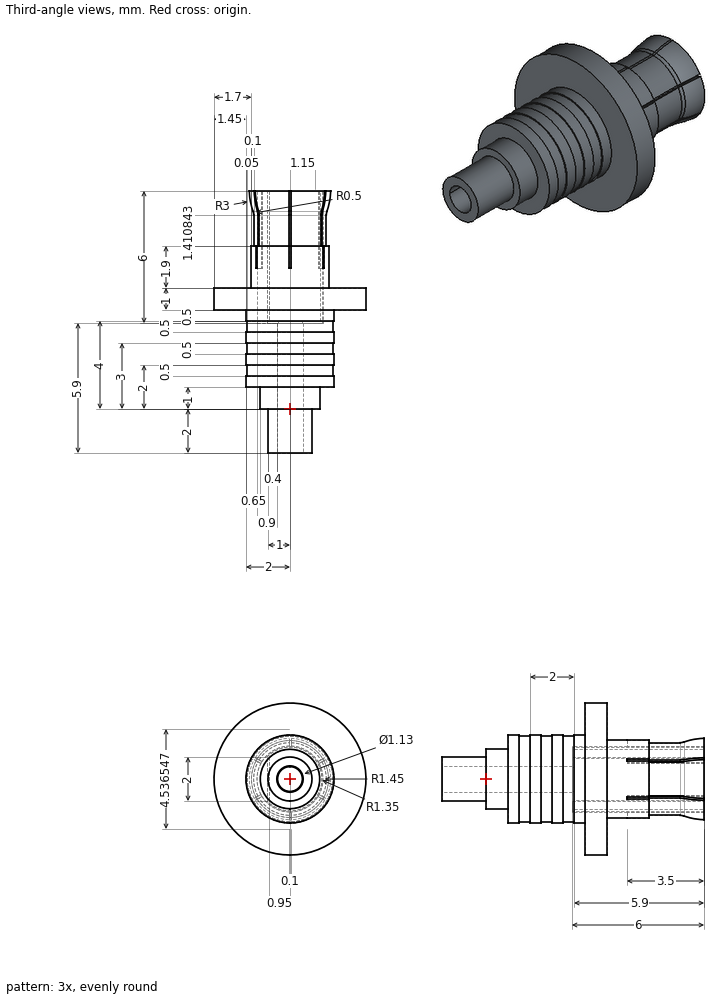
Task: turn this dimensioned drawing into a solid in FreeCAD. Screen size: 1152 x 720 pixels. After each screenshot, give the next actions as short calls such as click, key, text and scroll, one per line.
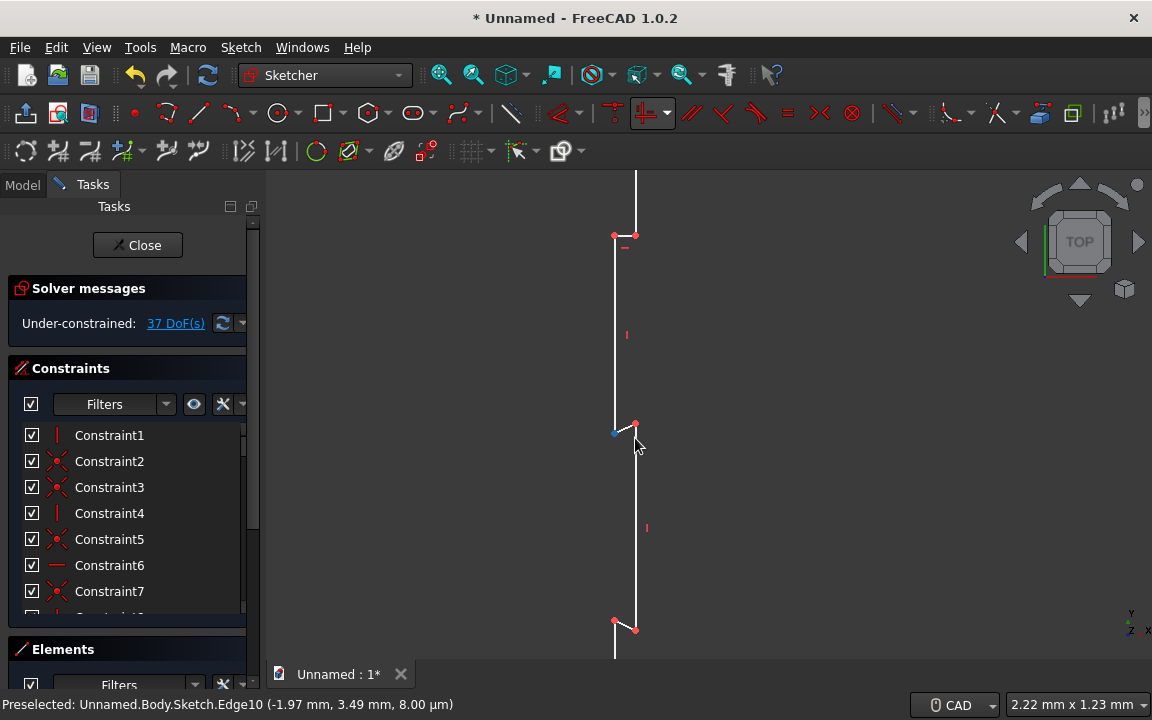
click(625, 429)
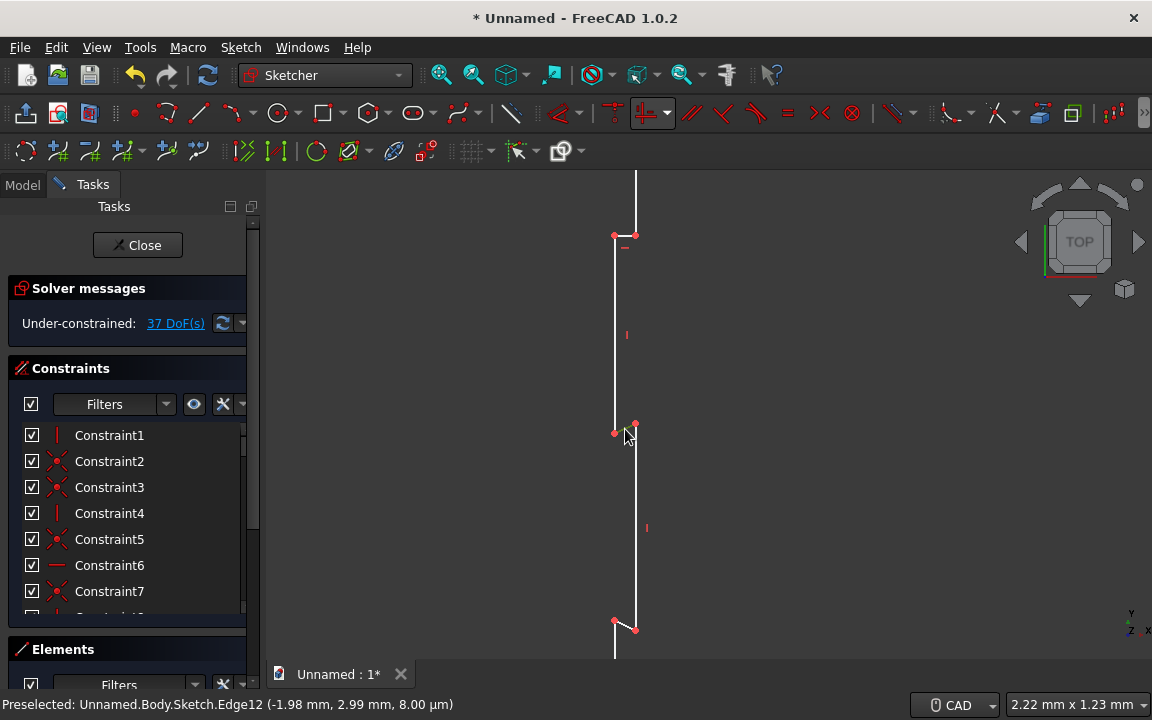
key(h)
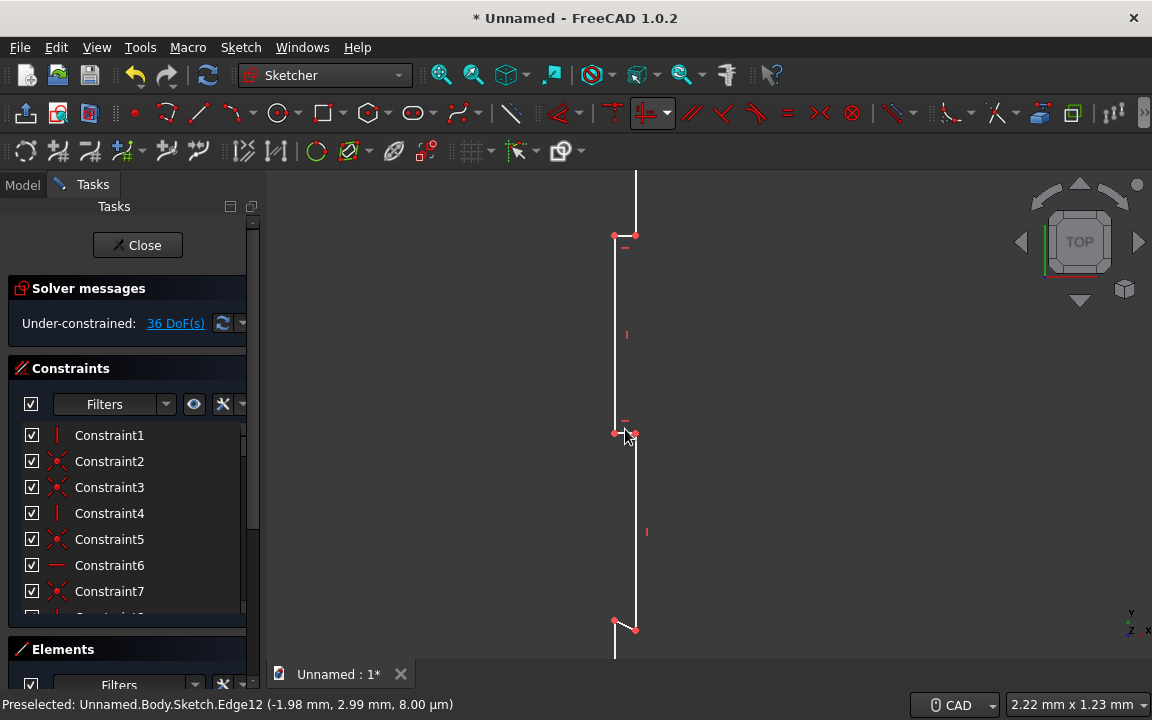
click(625, 626)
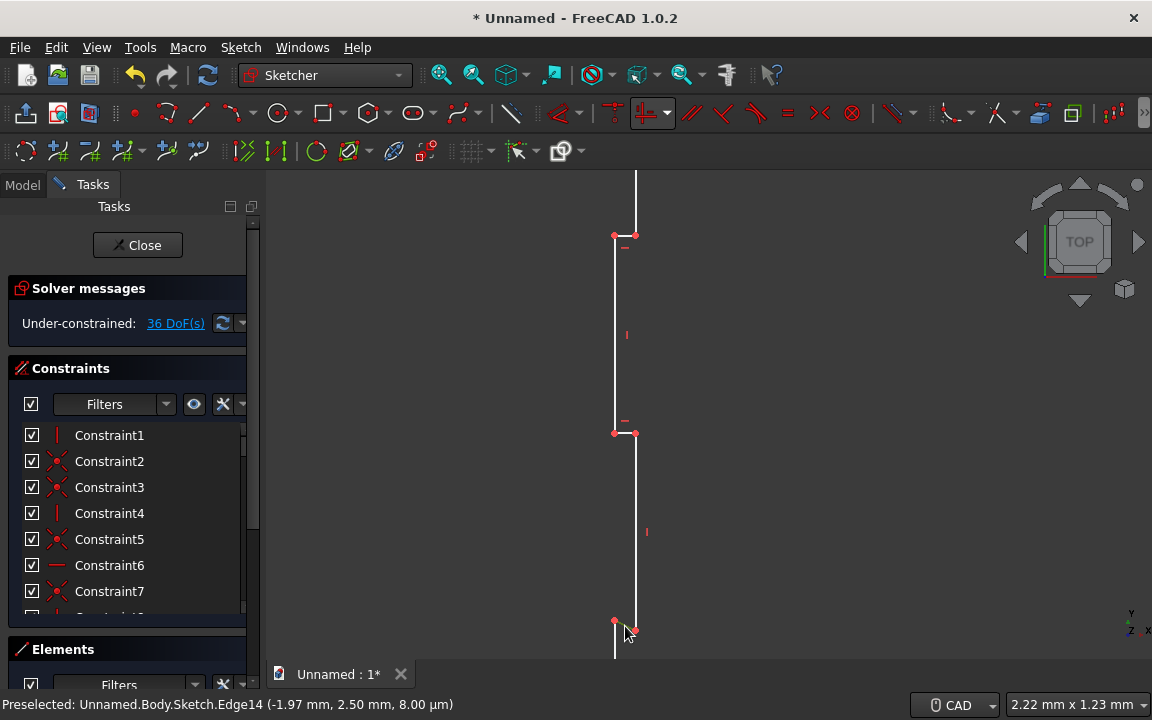
key(h)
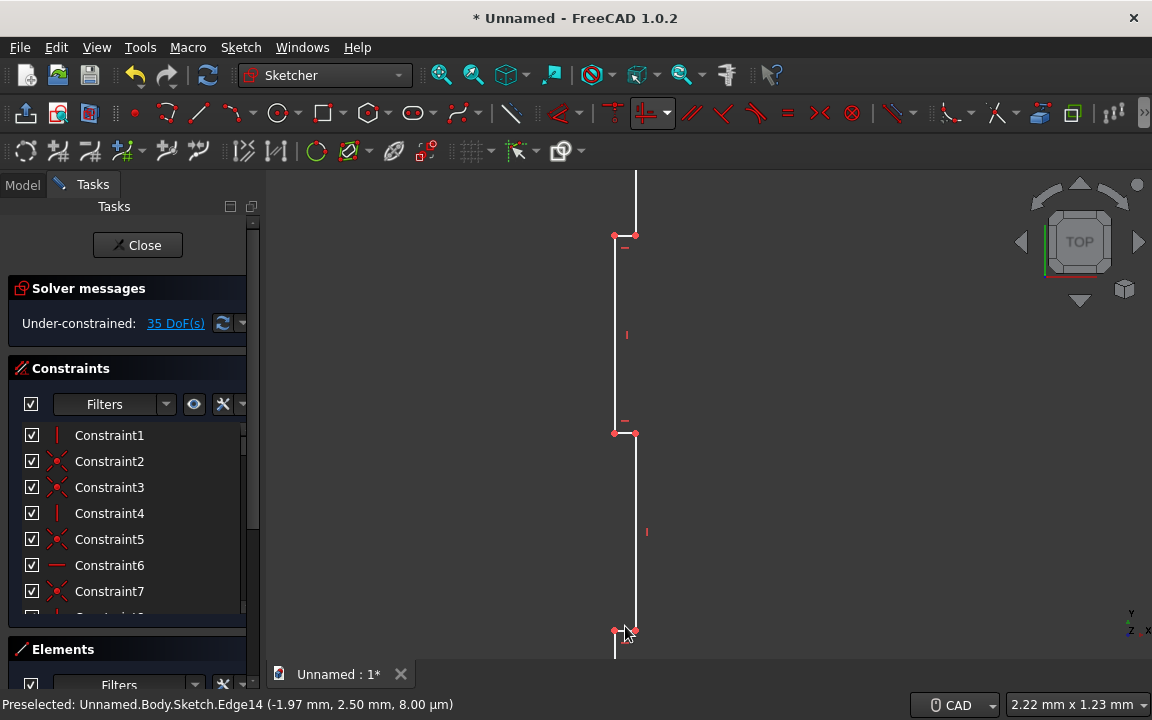
scroll(635, 438, down, 14)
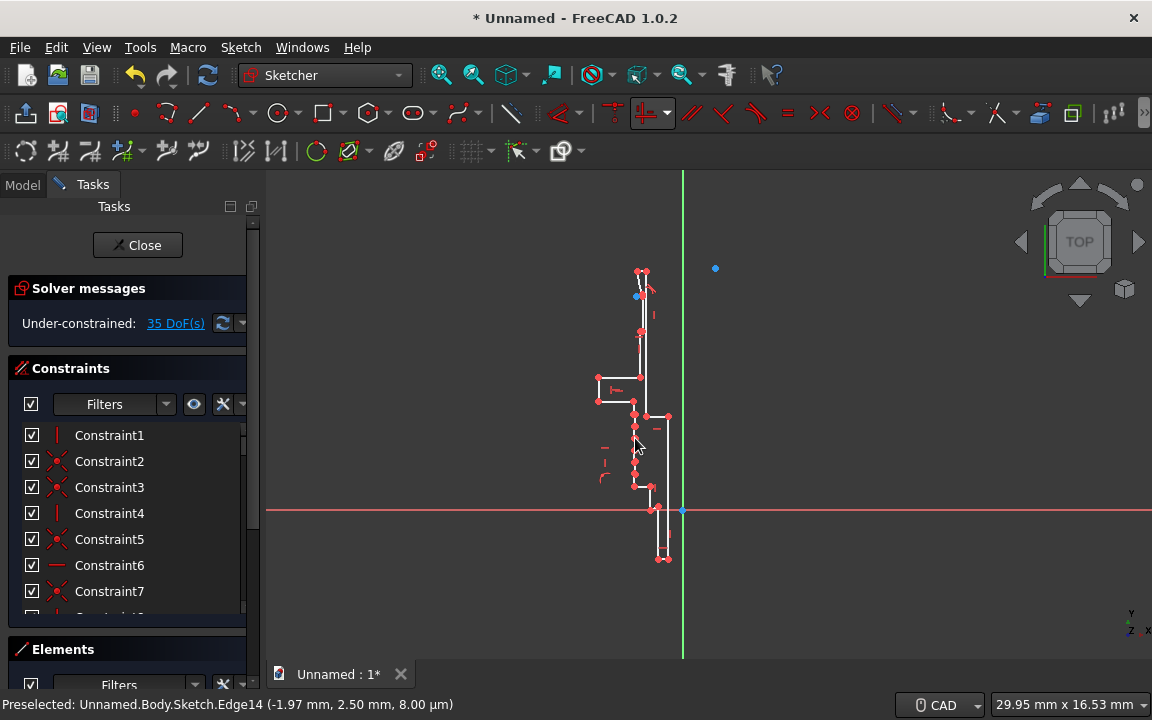
scroll(635, 462, up, 14)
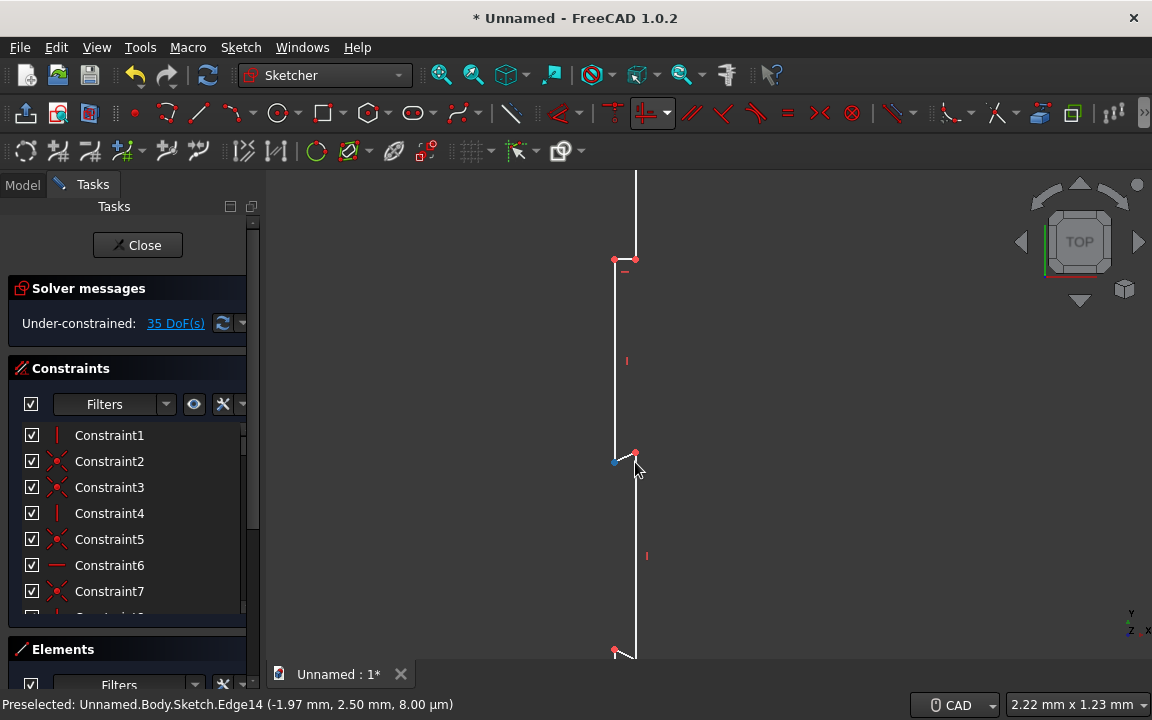
click(625, 457)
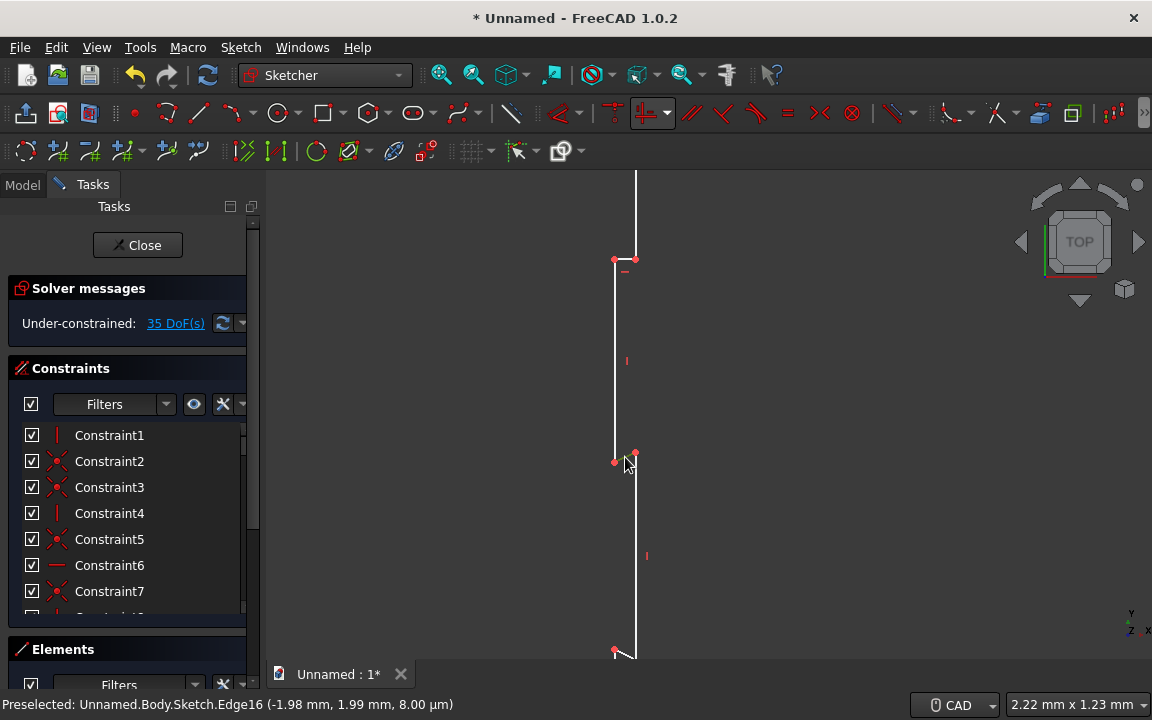
key(h)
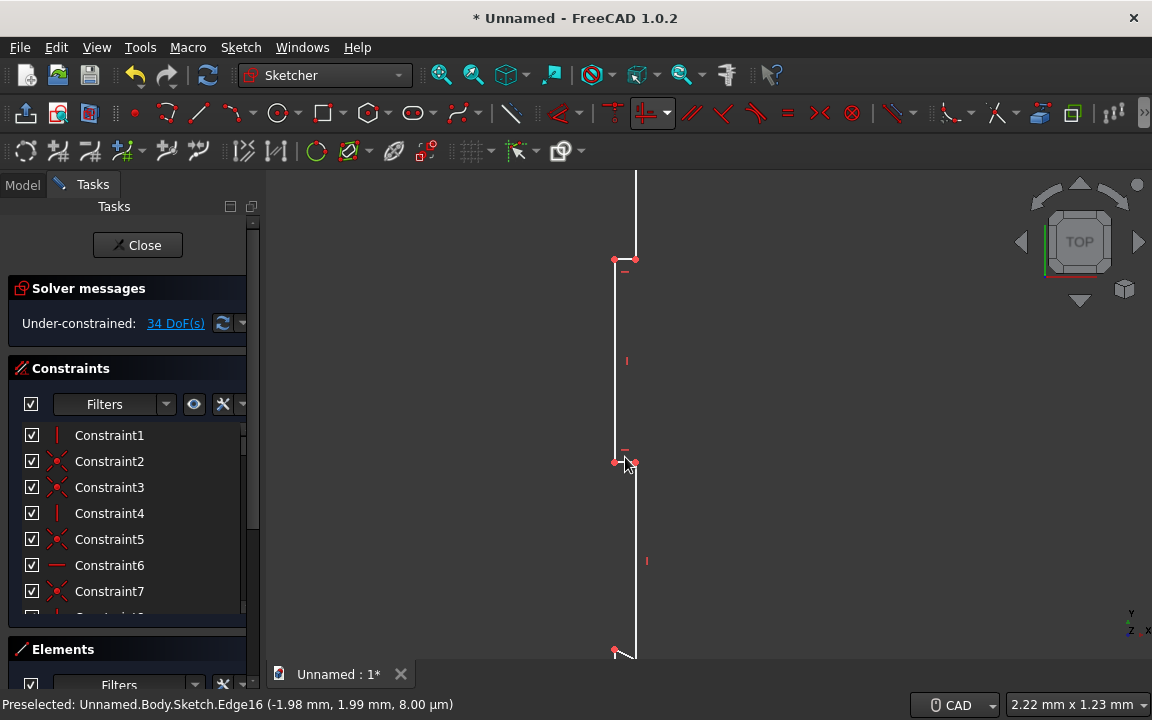
scroll(635, 462, down, 14)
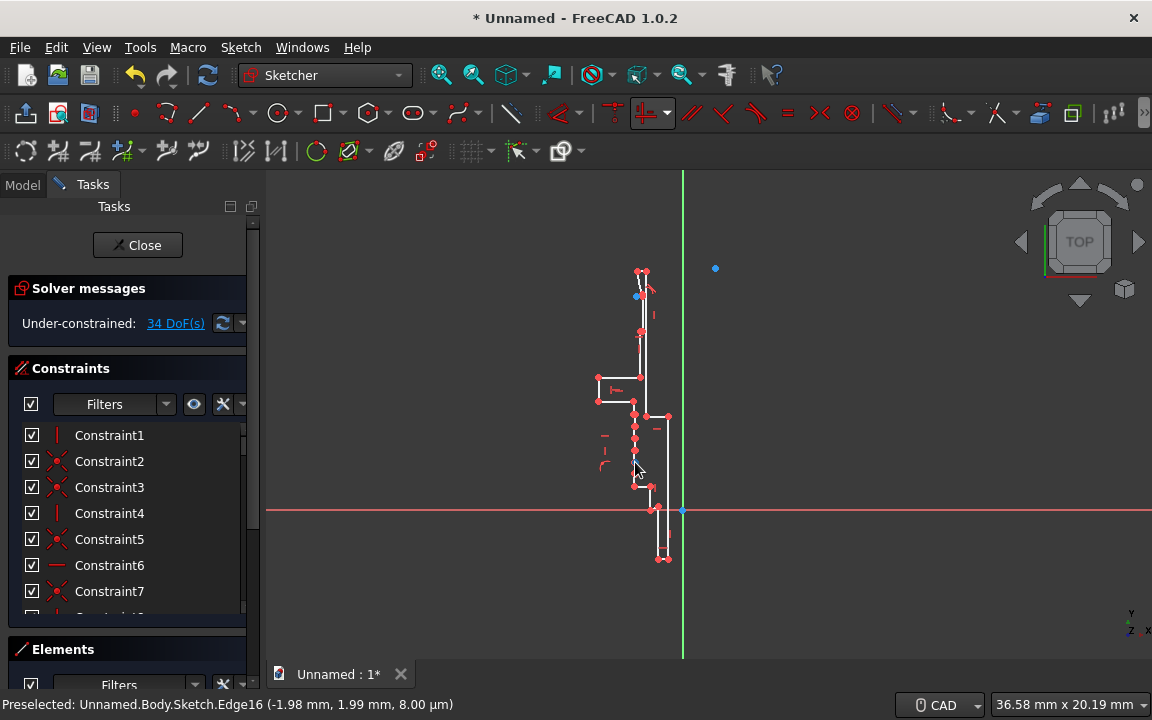
scroll(635, 474, up, 14)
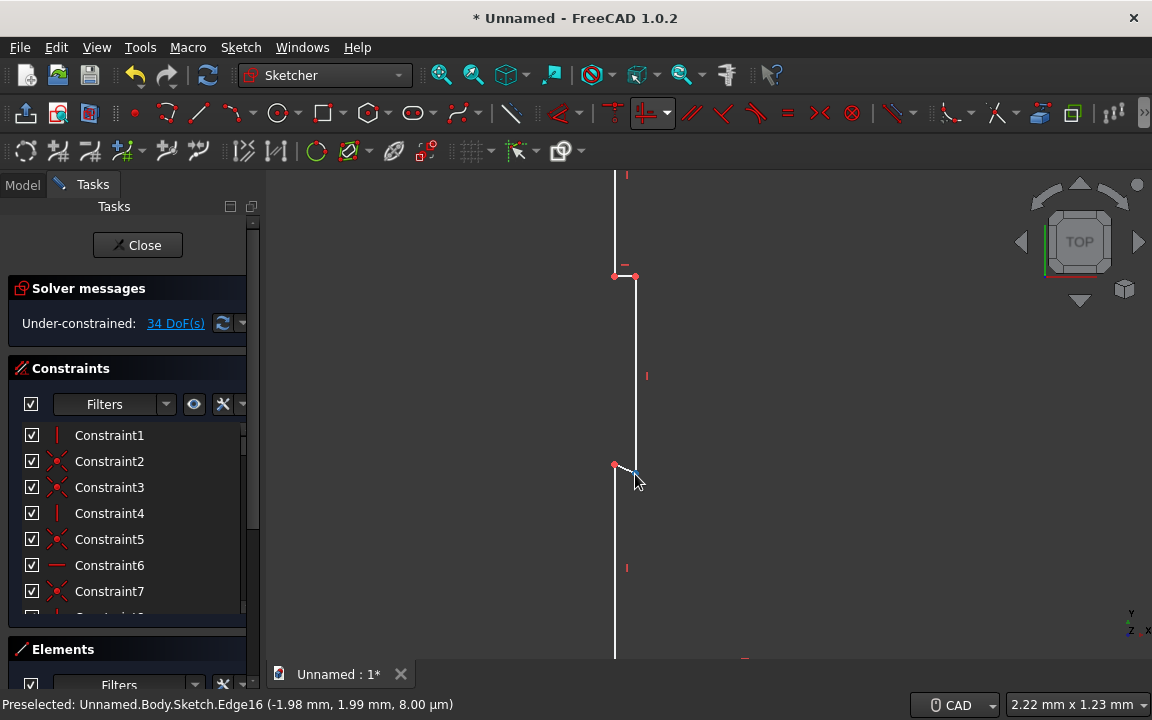
click(625, 469)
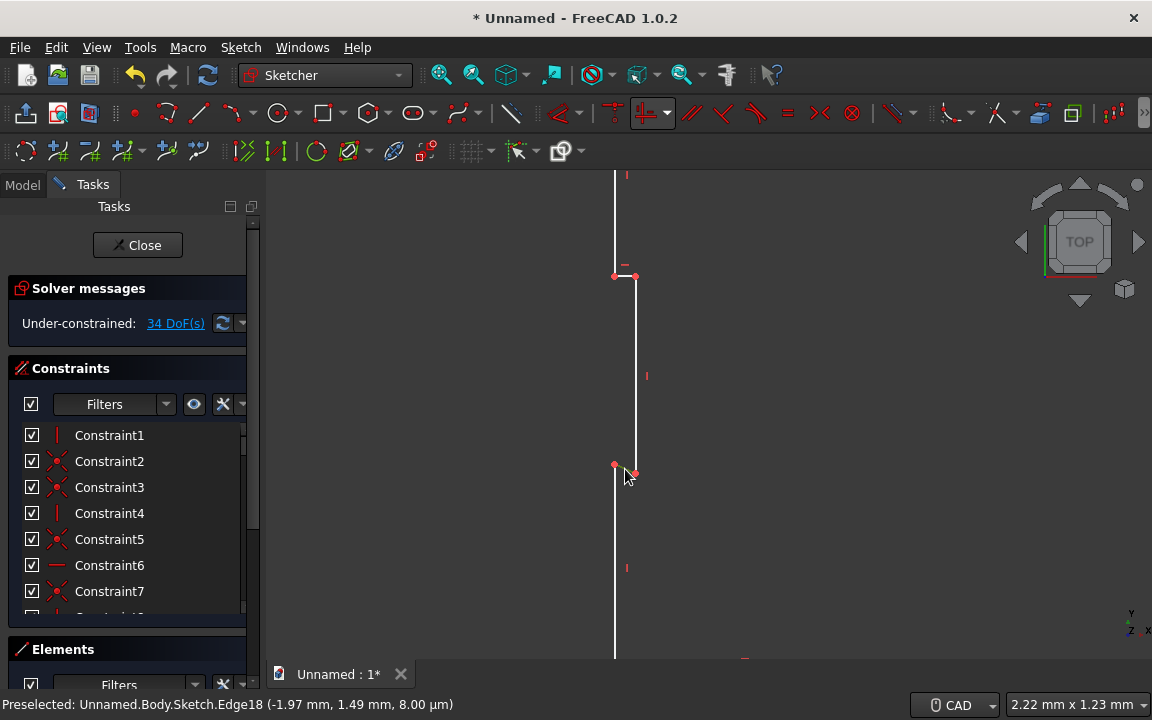
click(670, 114)